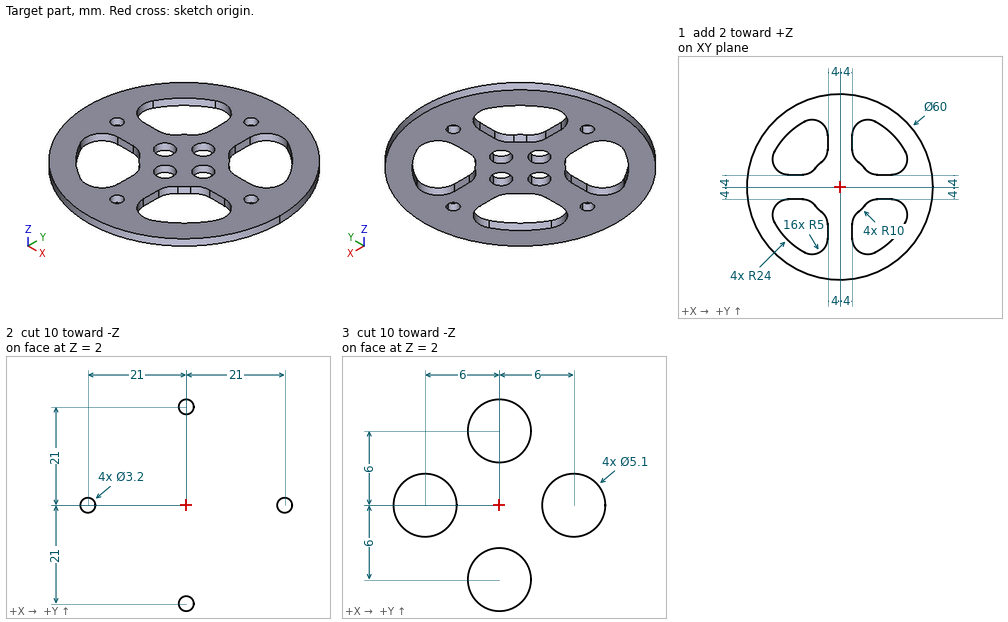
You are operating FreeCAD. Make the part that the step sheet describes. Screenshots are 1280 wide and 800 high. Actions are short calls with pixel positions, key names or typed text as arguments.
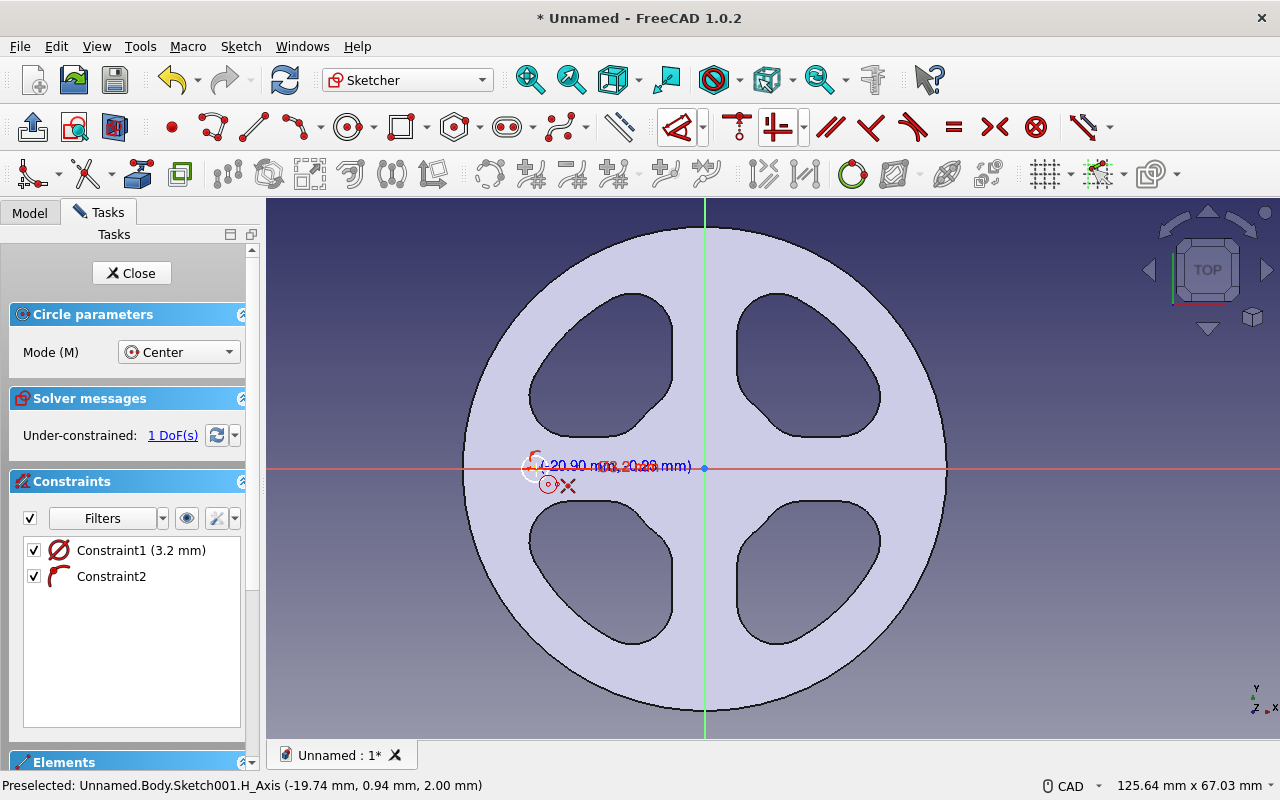
scroll(705, 299, up, 3)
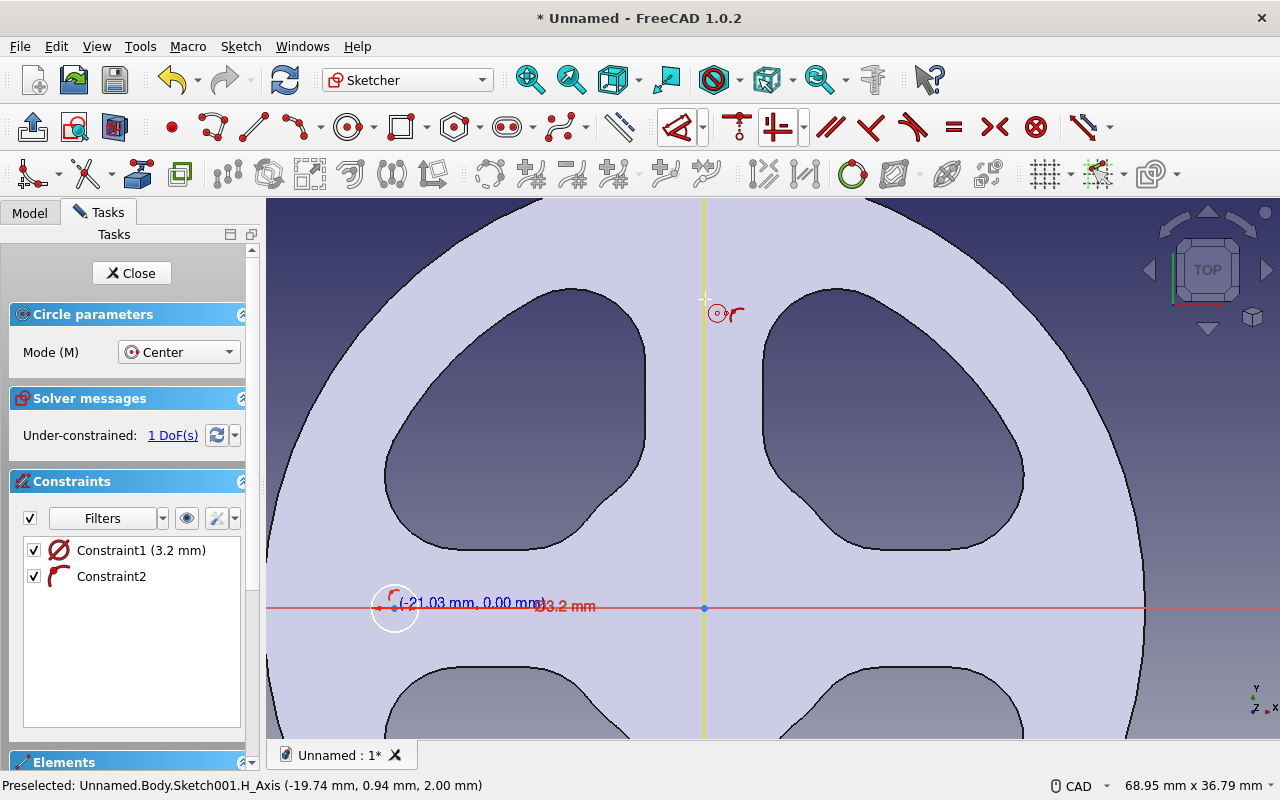
click(704, 300)
move(721, 283)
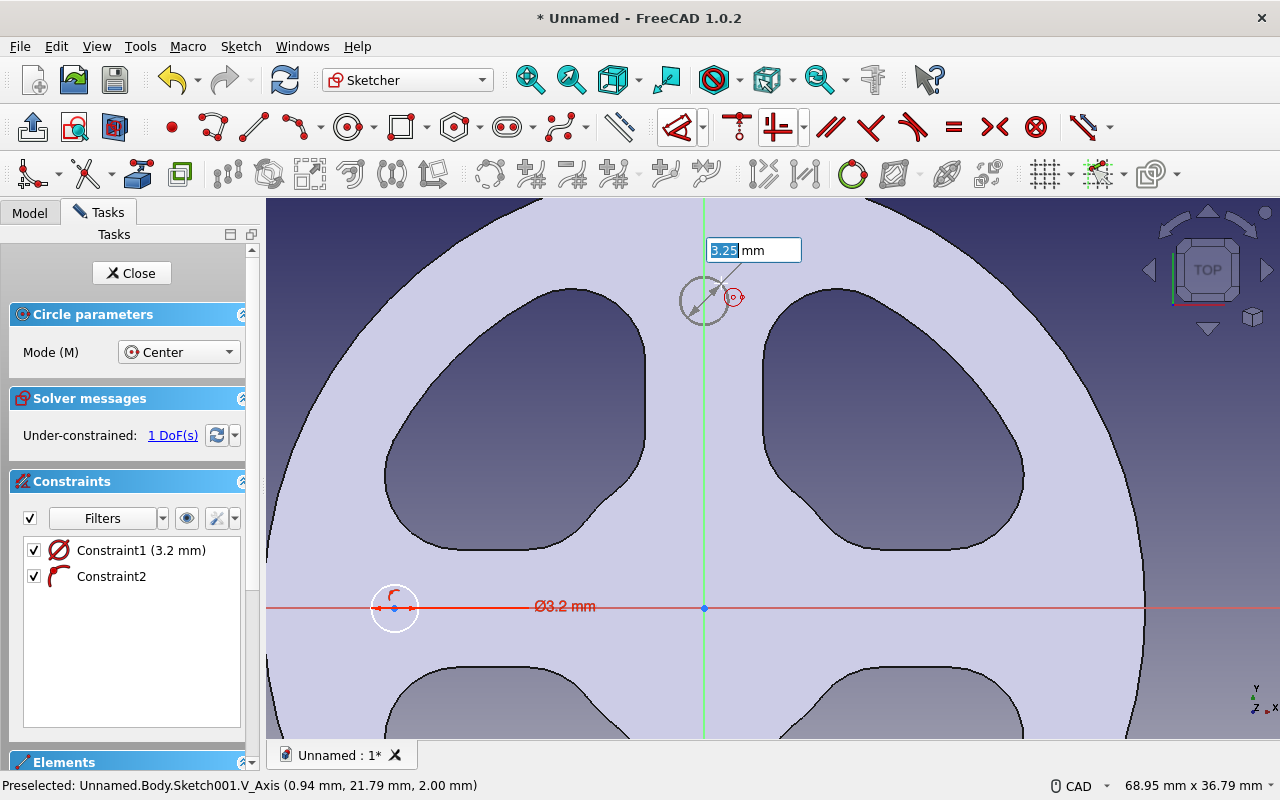
text(3.2)
key(Return)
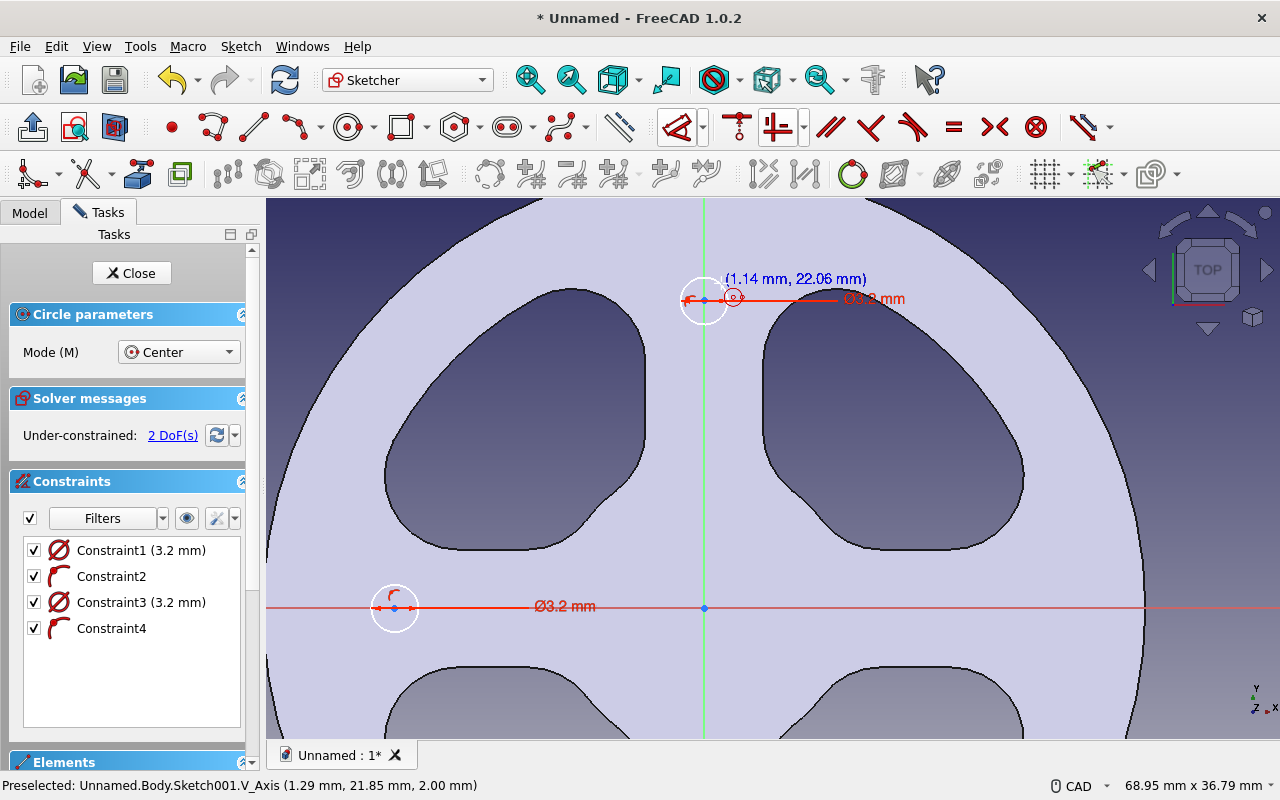
click(1013, 608)
move(1030, 592)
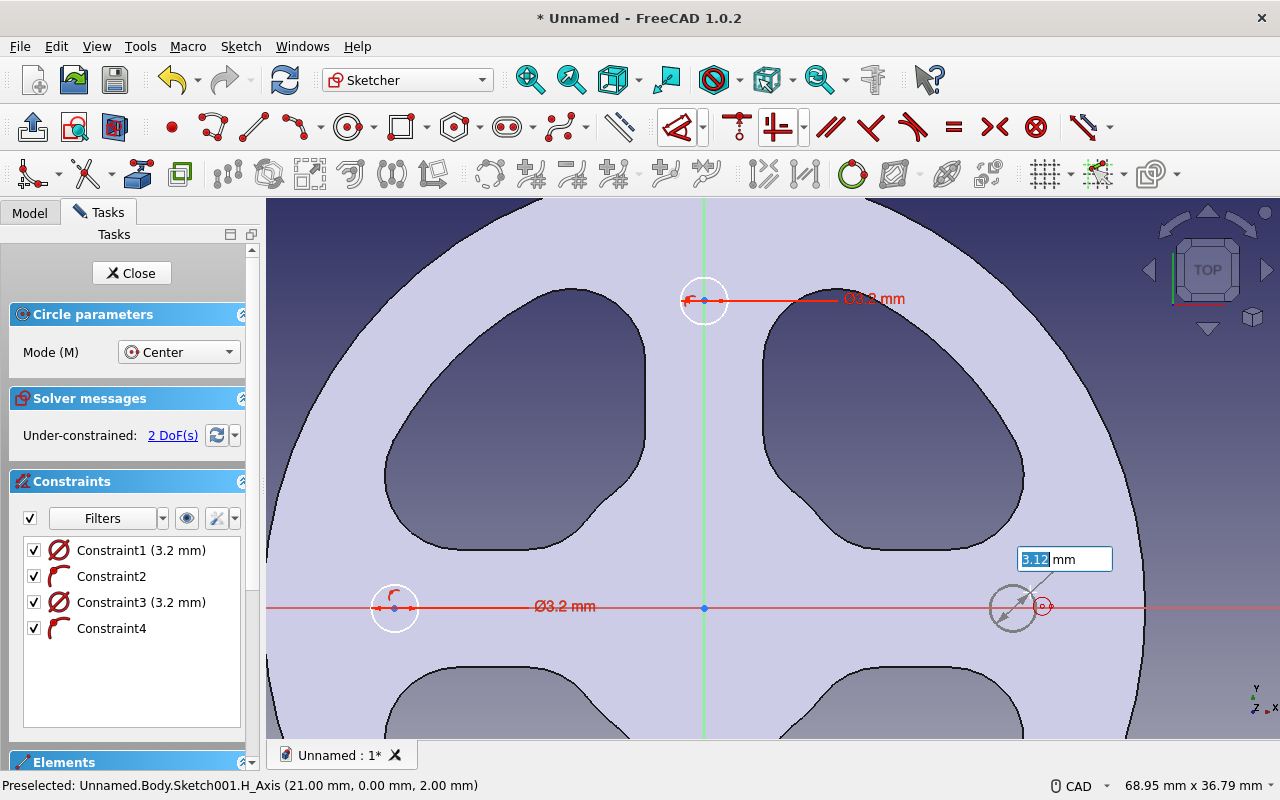
text(3.2)
key(Return)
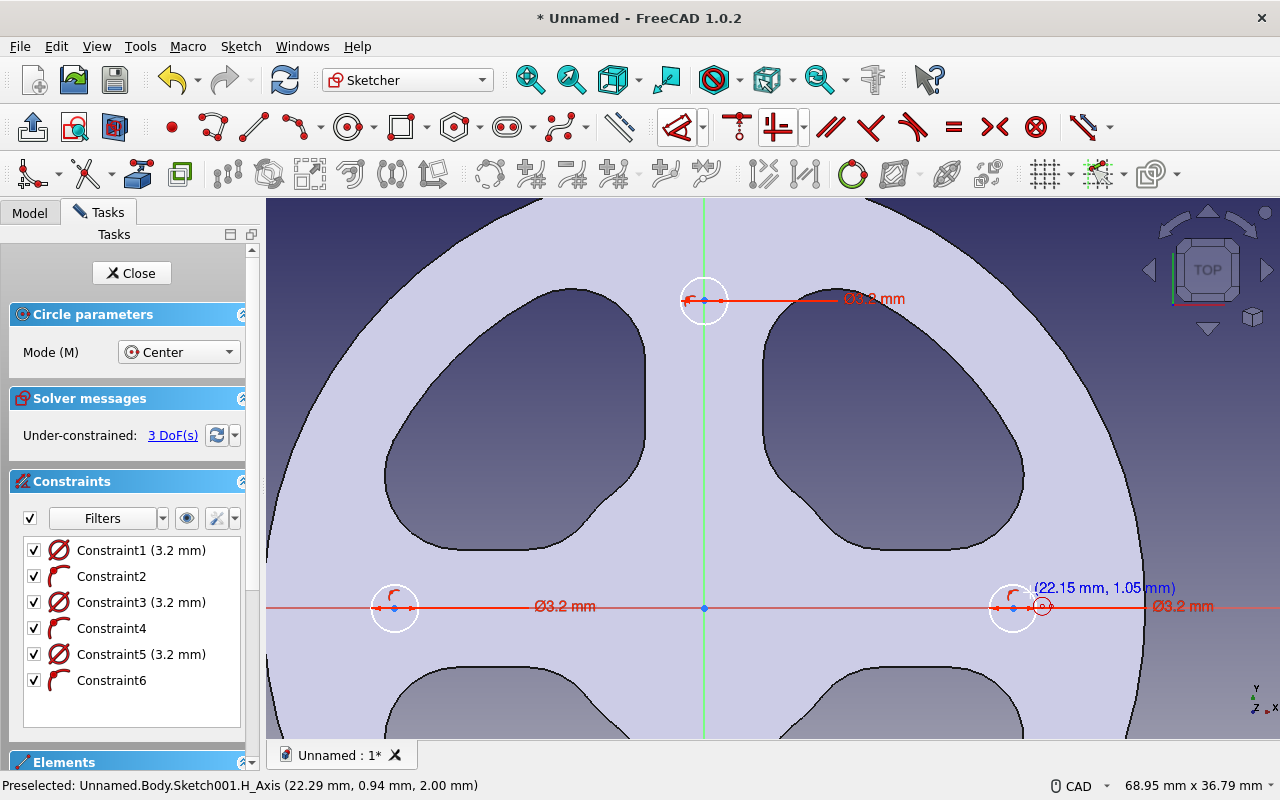
scroll(705, 298, down, 3)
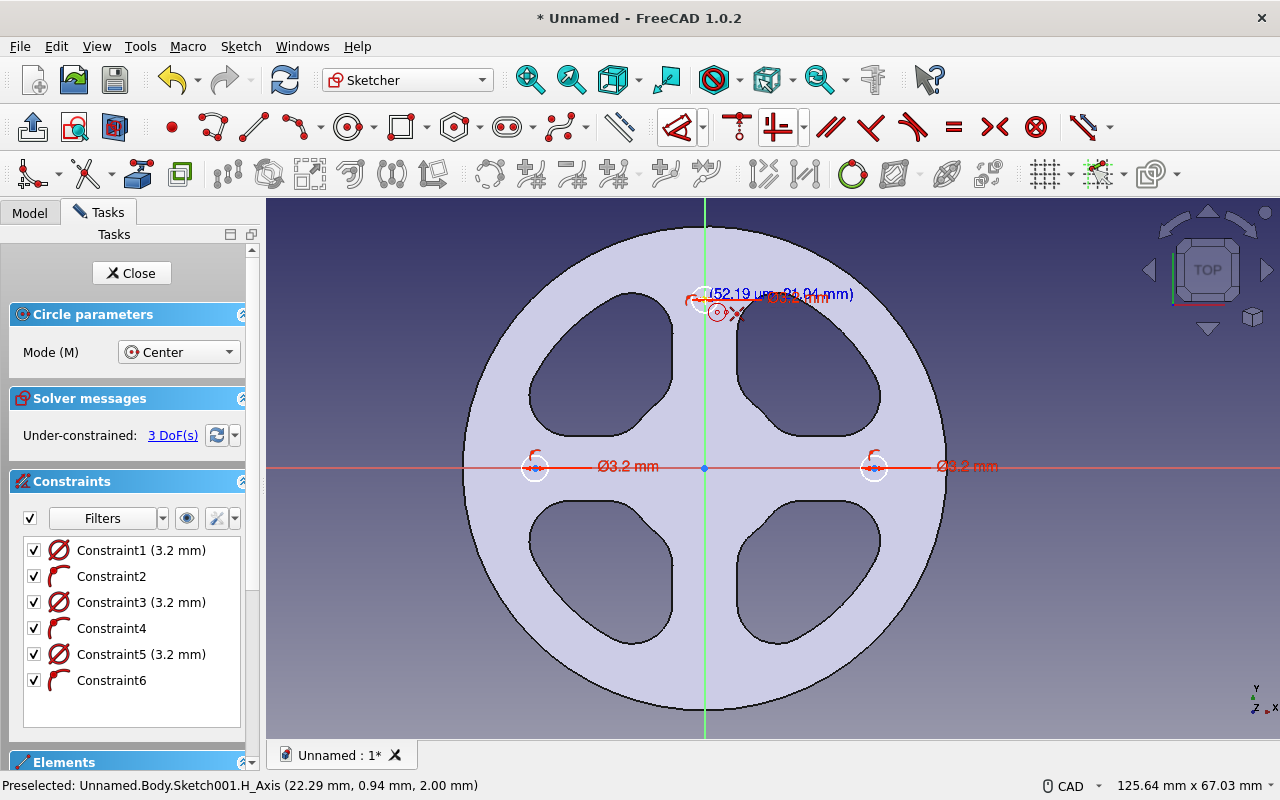
scroll(705, 638, up, 3)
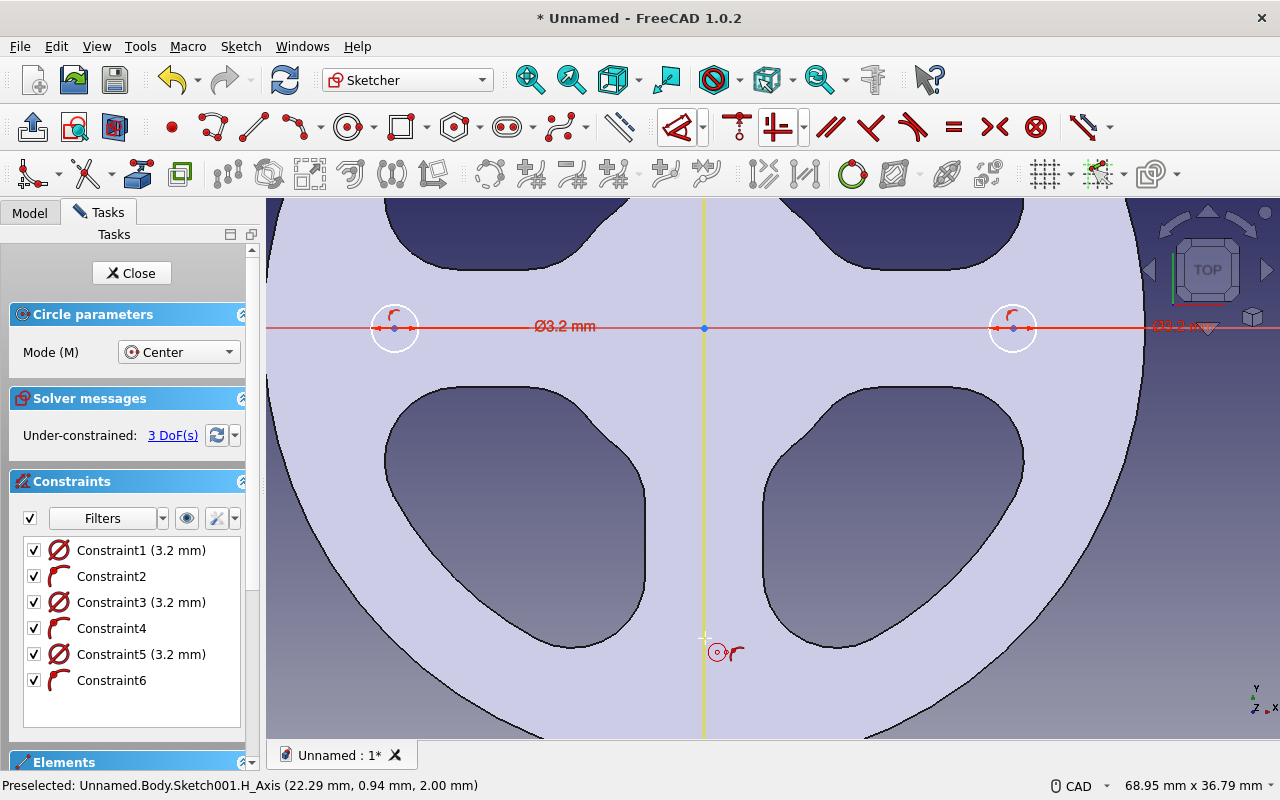
click(704, 637)
move(721, 621)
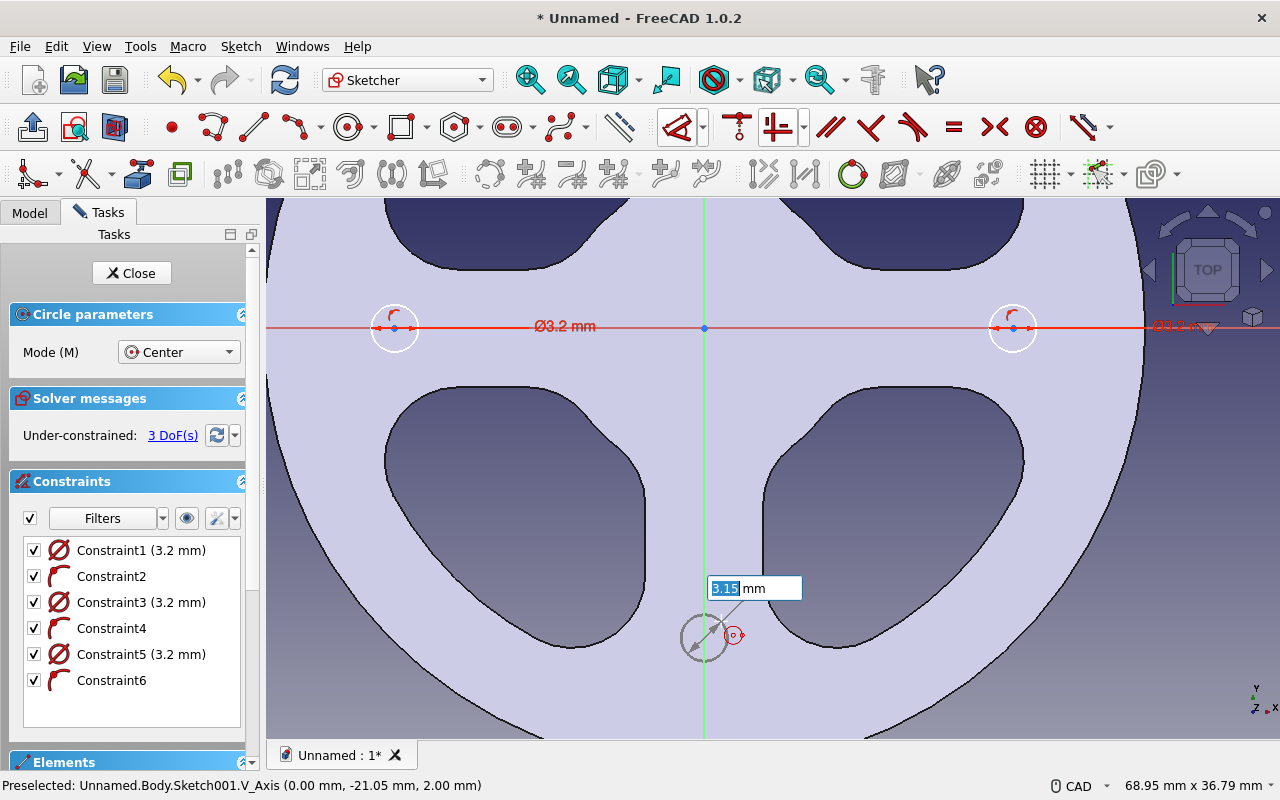
text(3.2)
key(Return)
key(Escape)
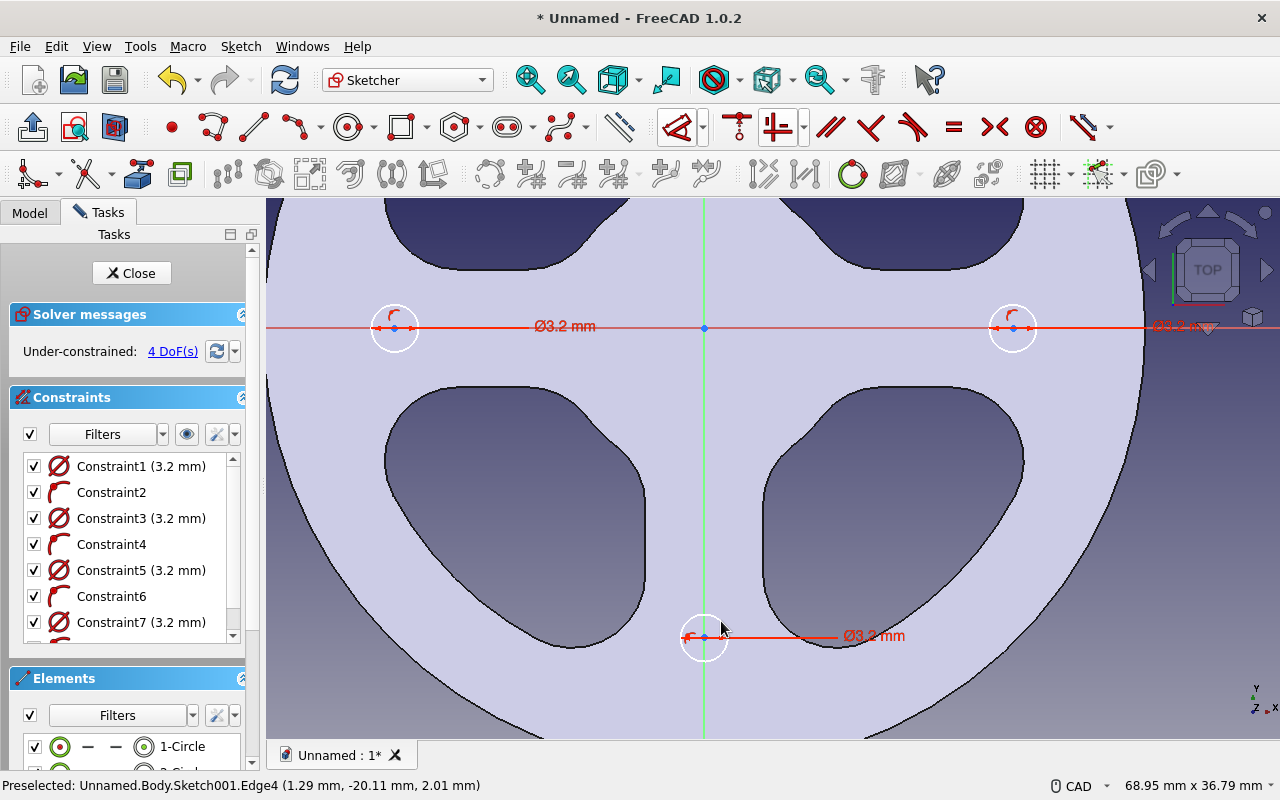
click(395, 328)